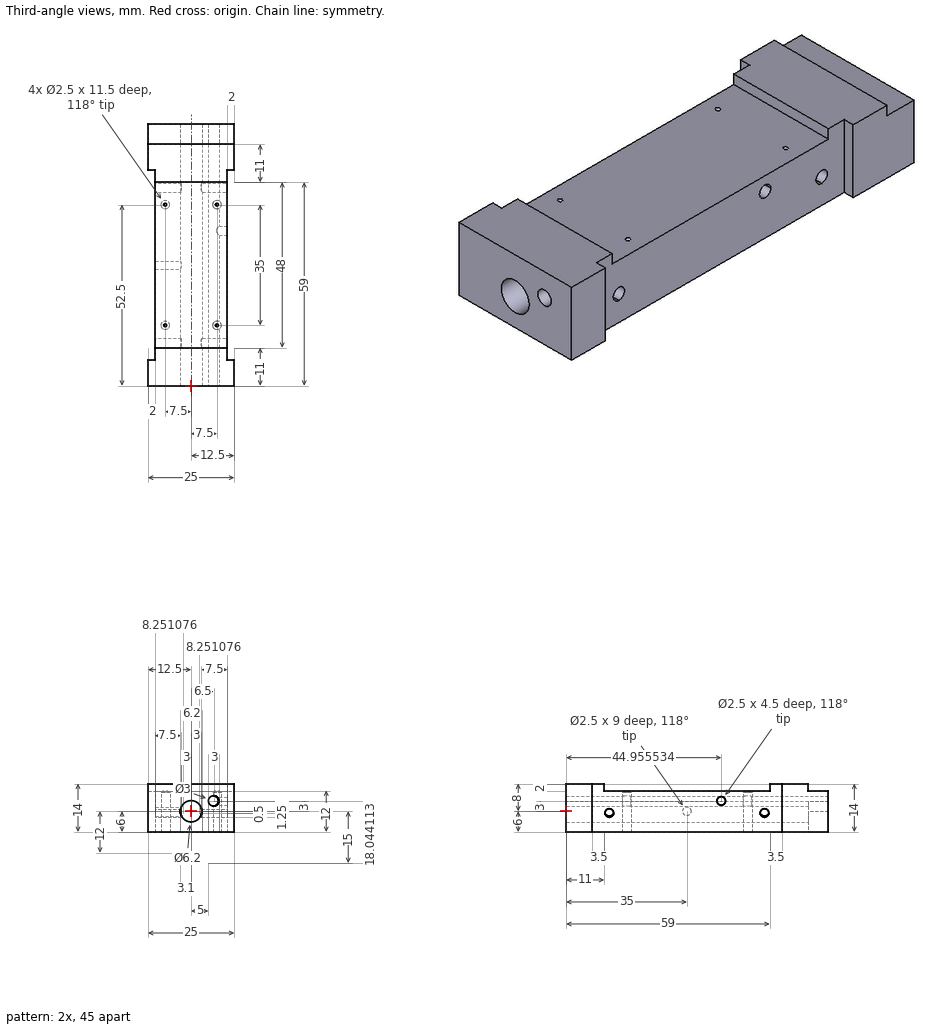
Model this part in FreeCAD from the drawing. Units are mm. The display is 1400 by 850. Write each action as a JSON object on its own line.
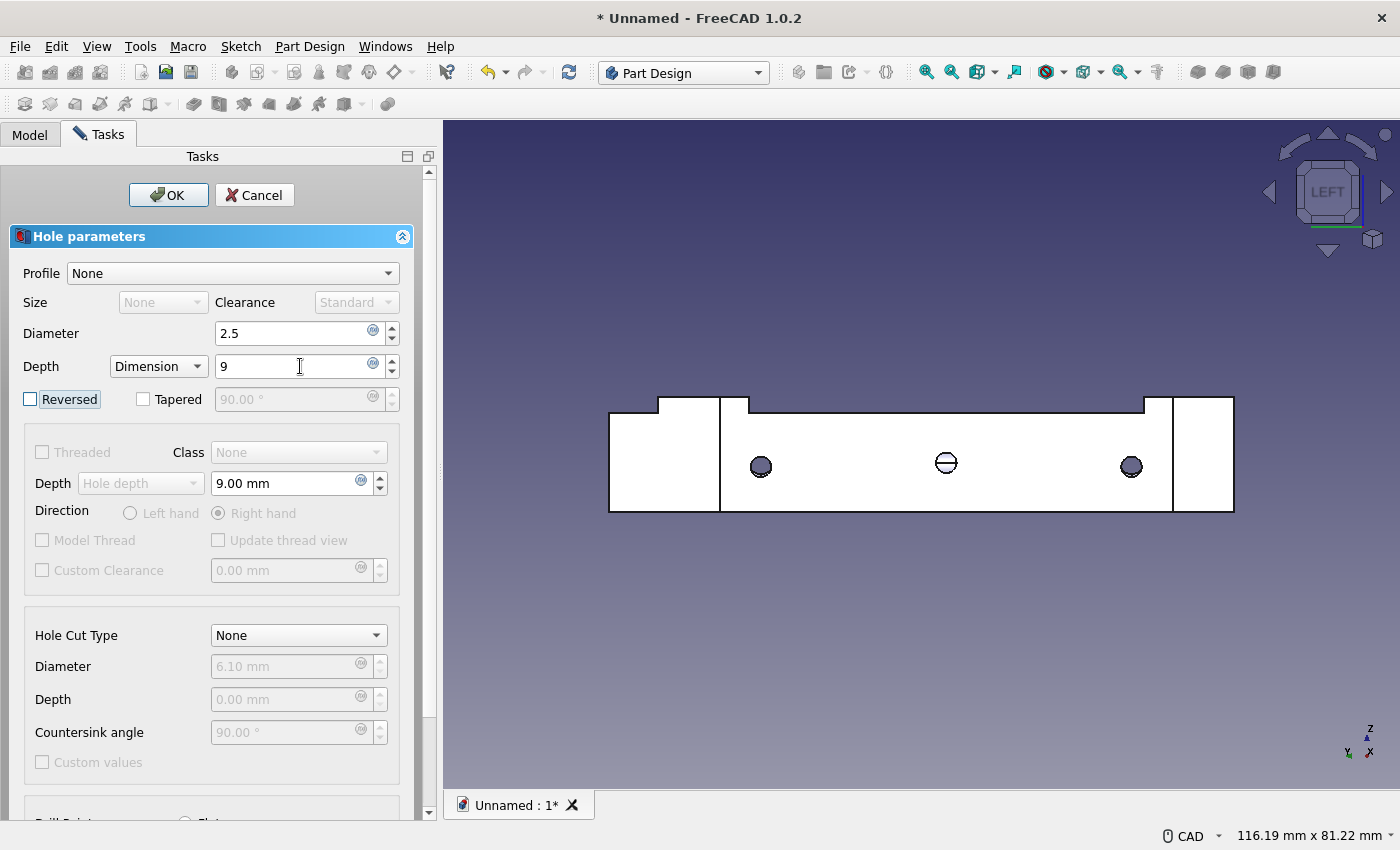
{"action": "left_click", "coordinate": [169, 195]}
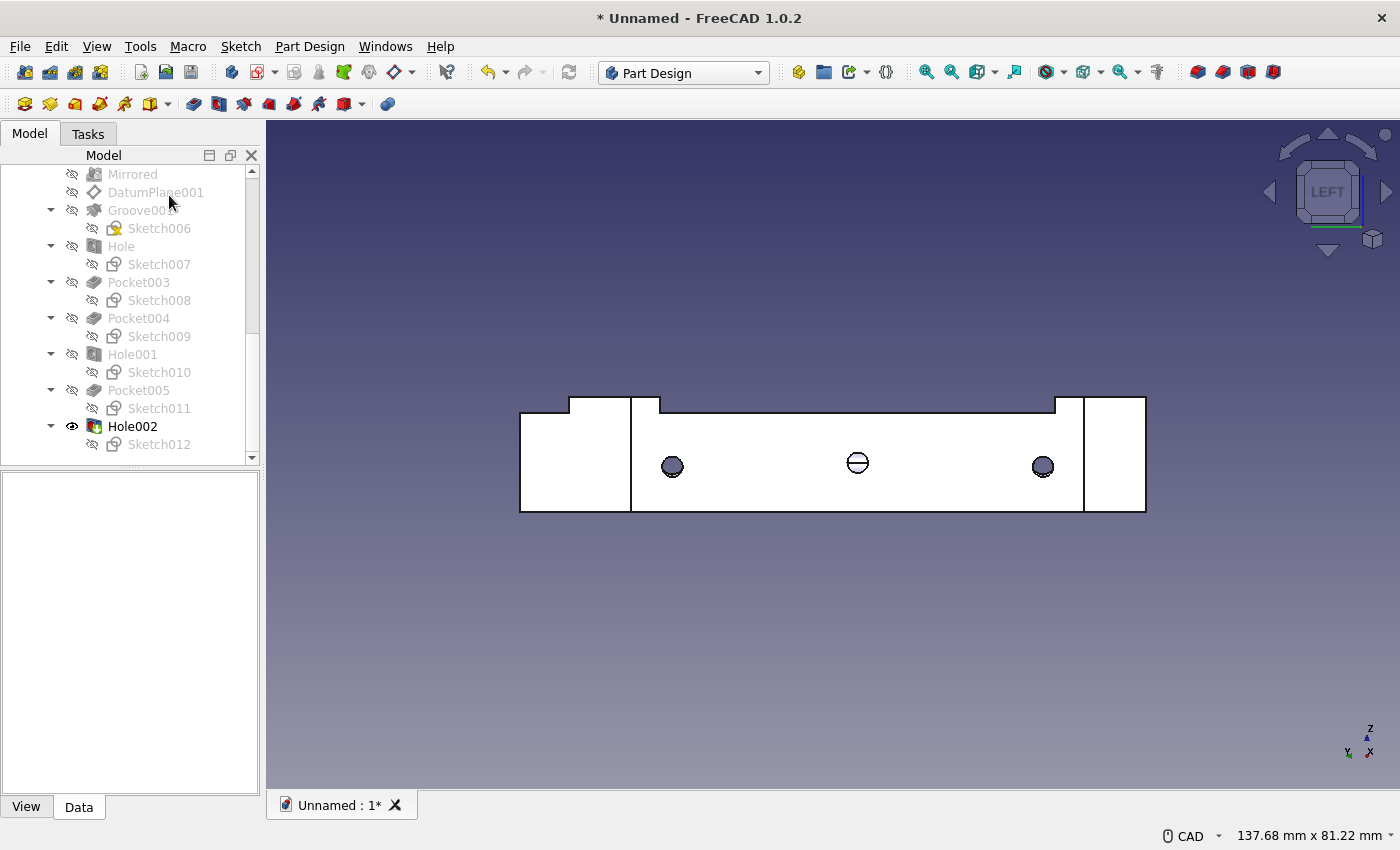
{"action": "key", "text": "0"}